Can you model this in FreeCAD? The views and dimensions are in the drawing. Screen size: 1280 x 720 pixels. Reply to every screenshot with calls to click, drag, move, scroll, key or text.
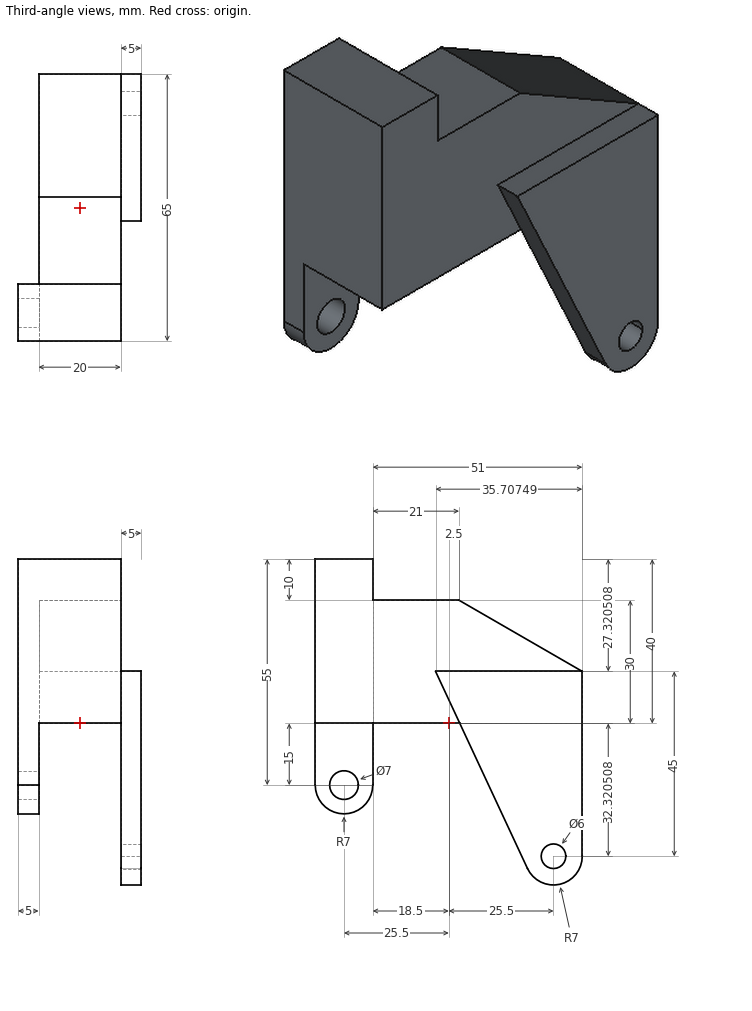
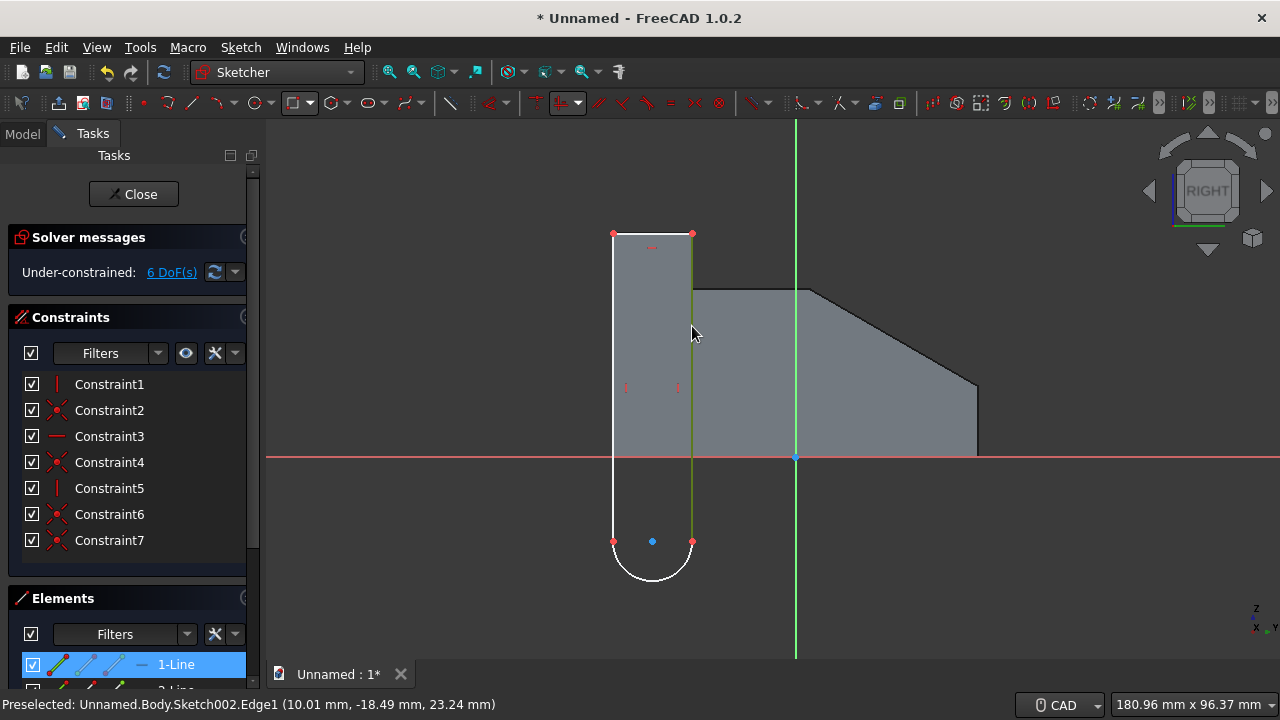
click(629, 574)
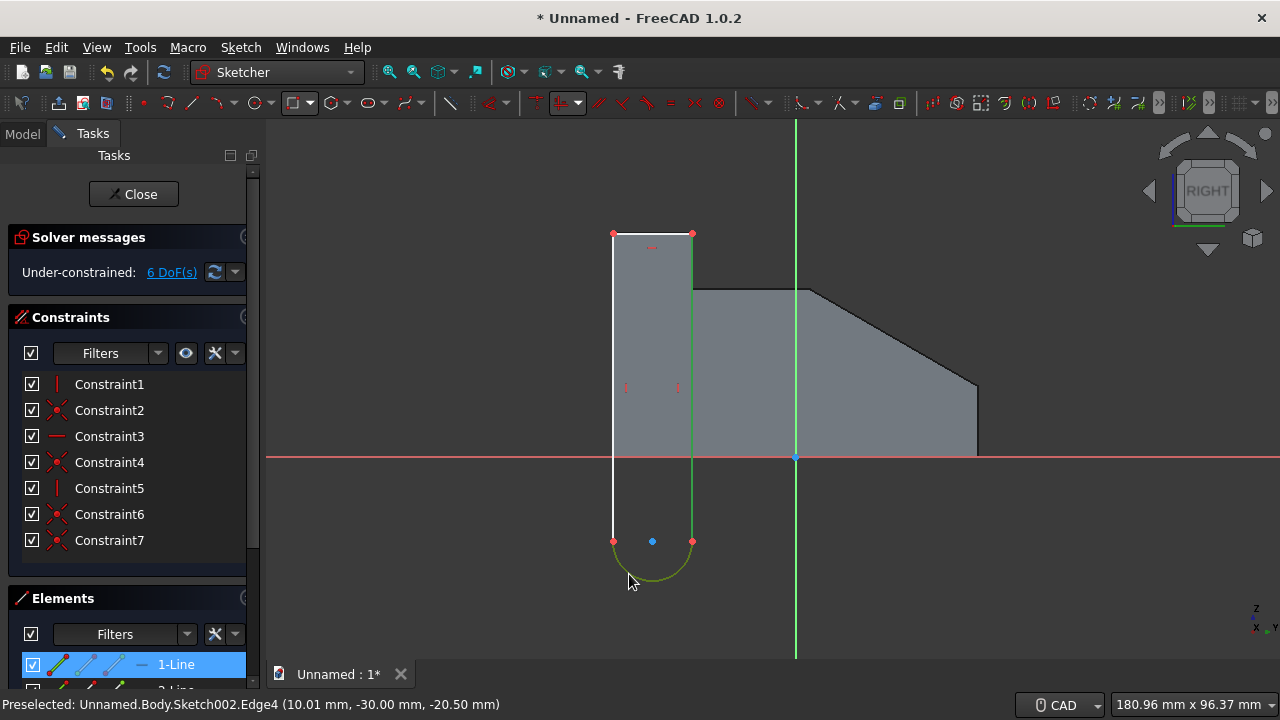
key(t)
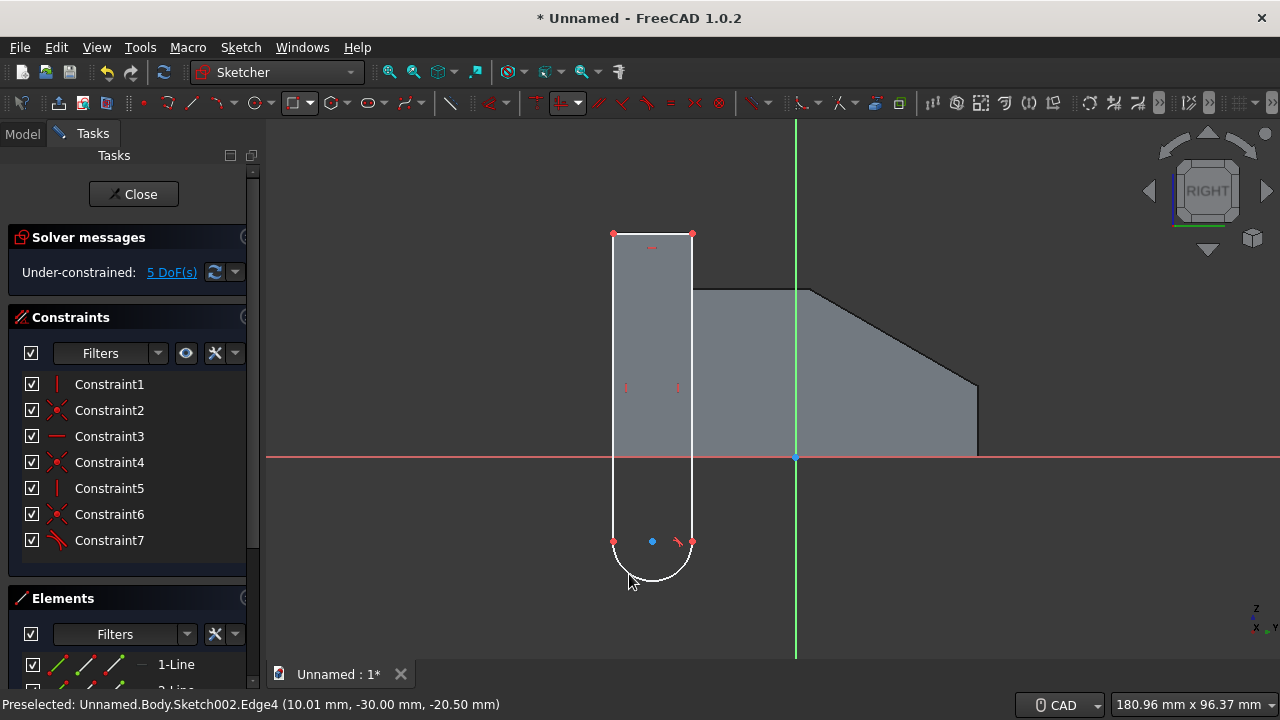
click(613, 326)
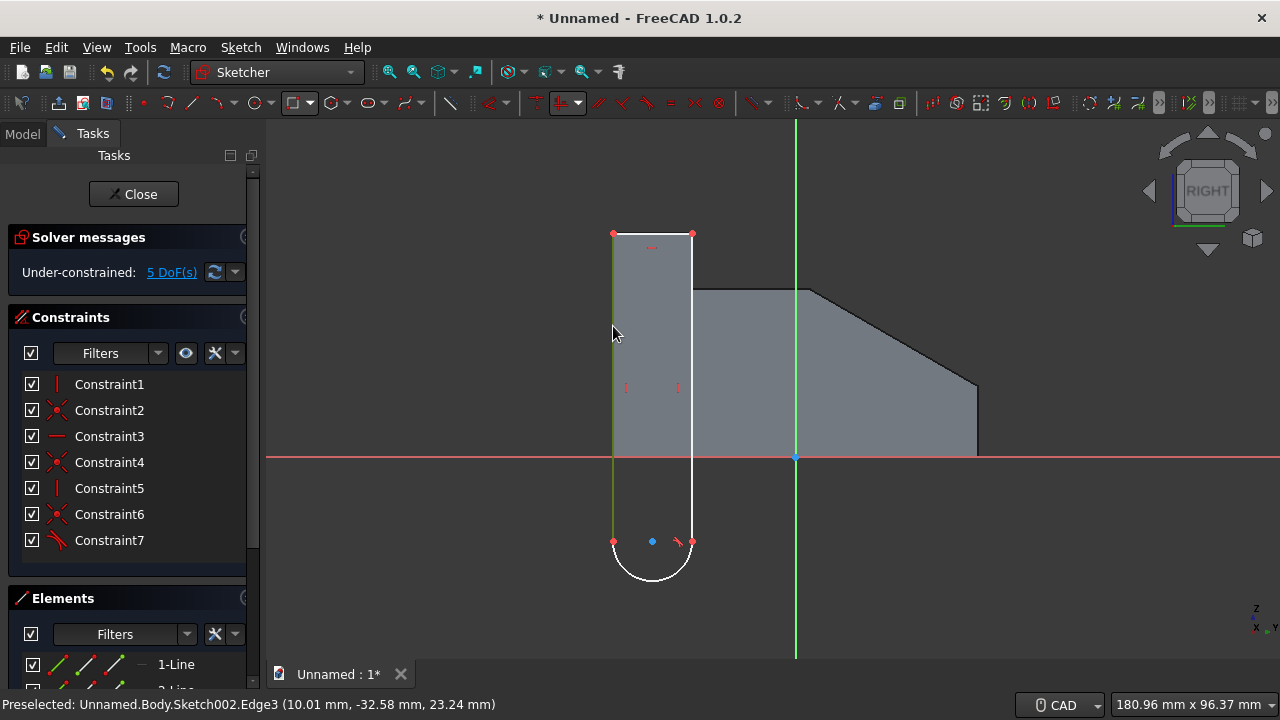
click(630, 574)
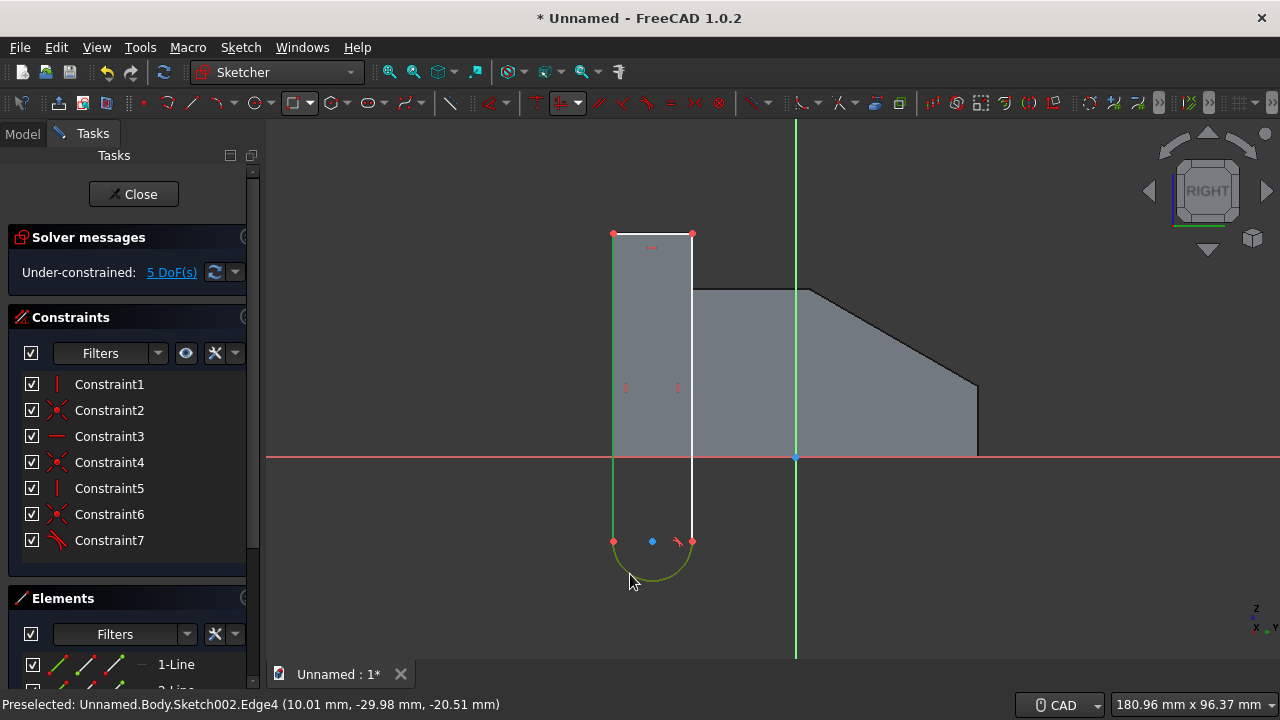
key(t)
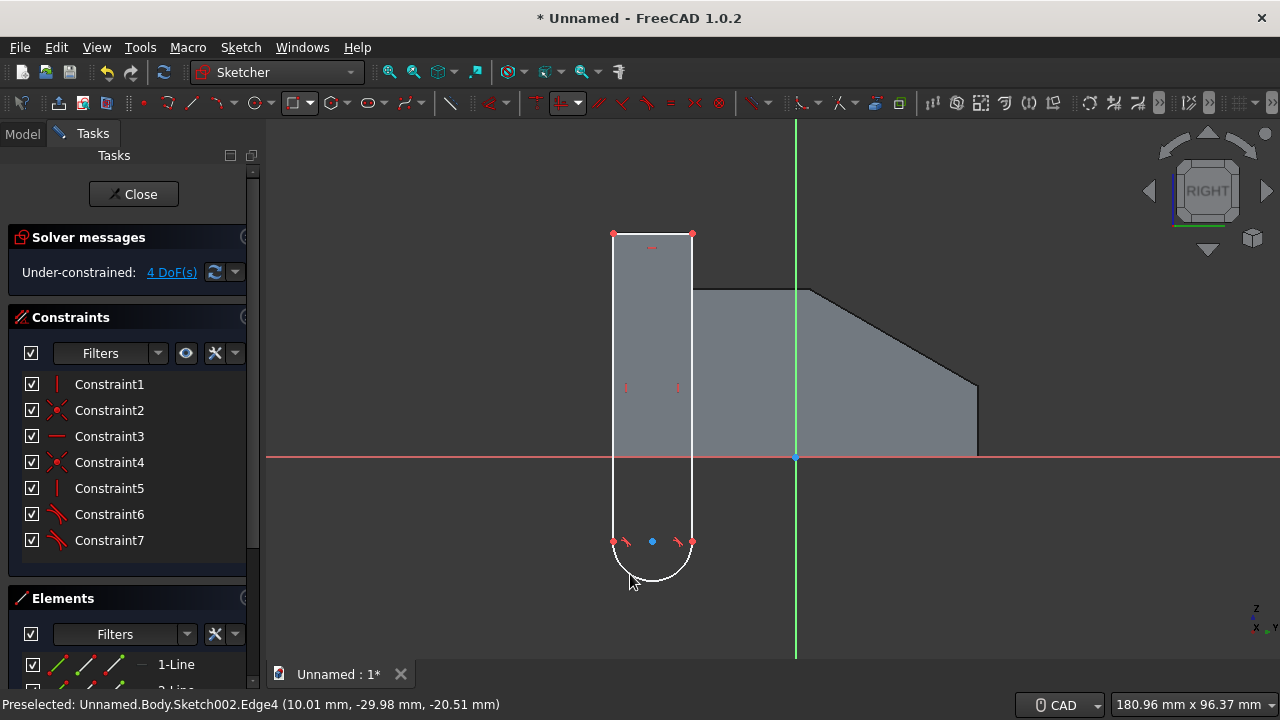
key(d)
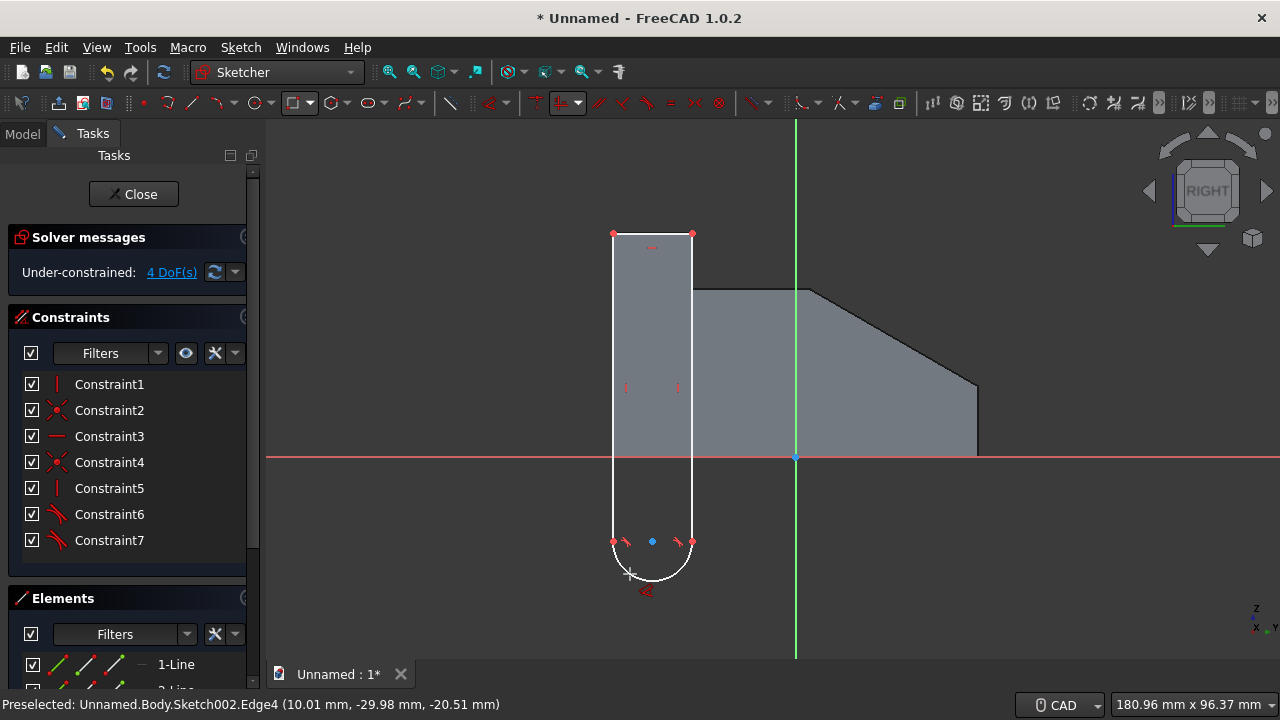
click(629, 573)
click(610, 599)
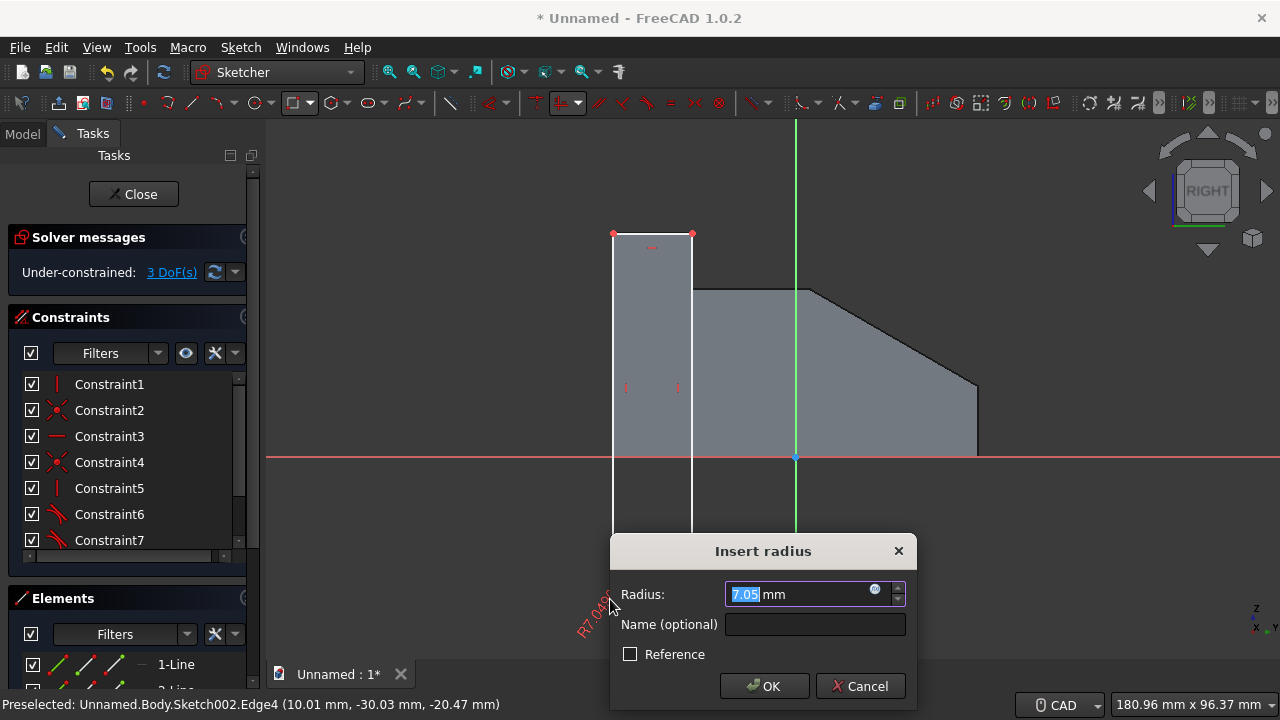
text(7)
key(Return)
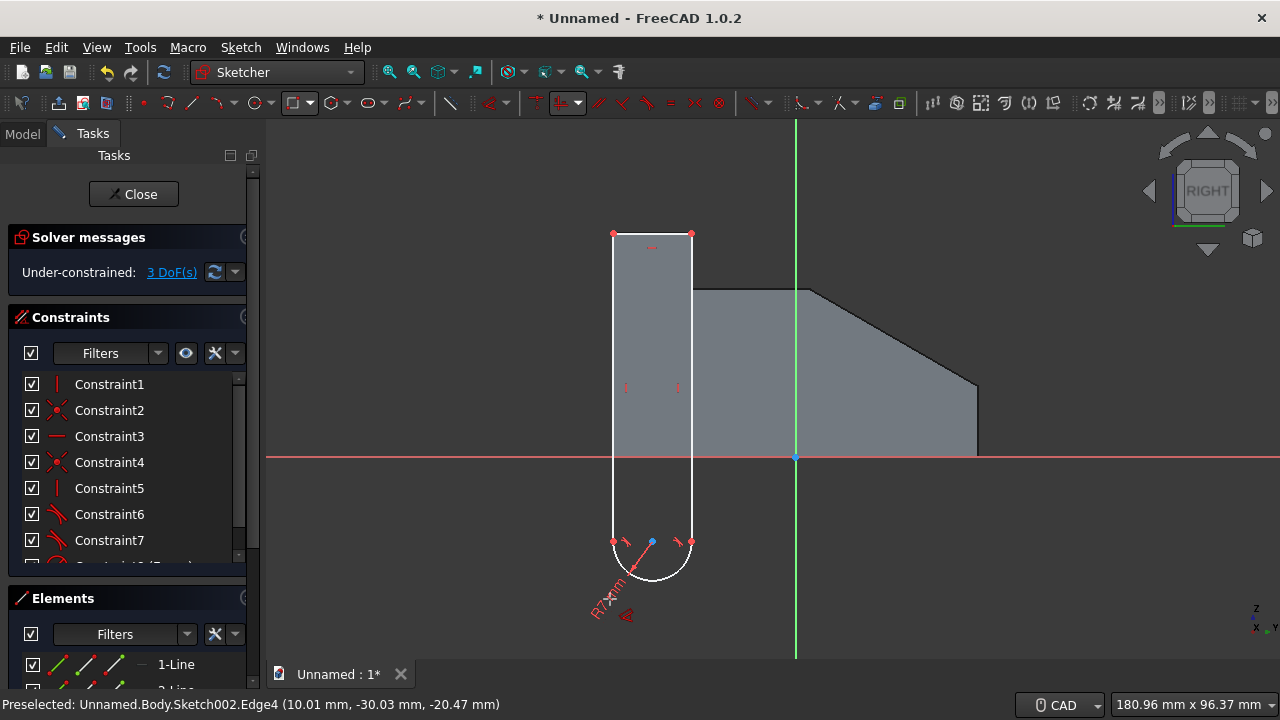
click(692, 326)
click(658, 388)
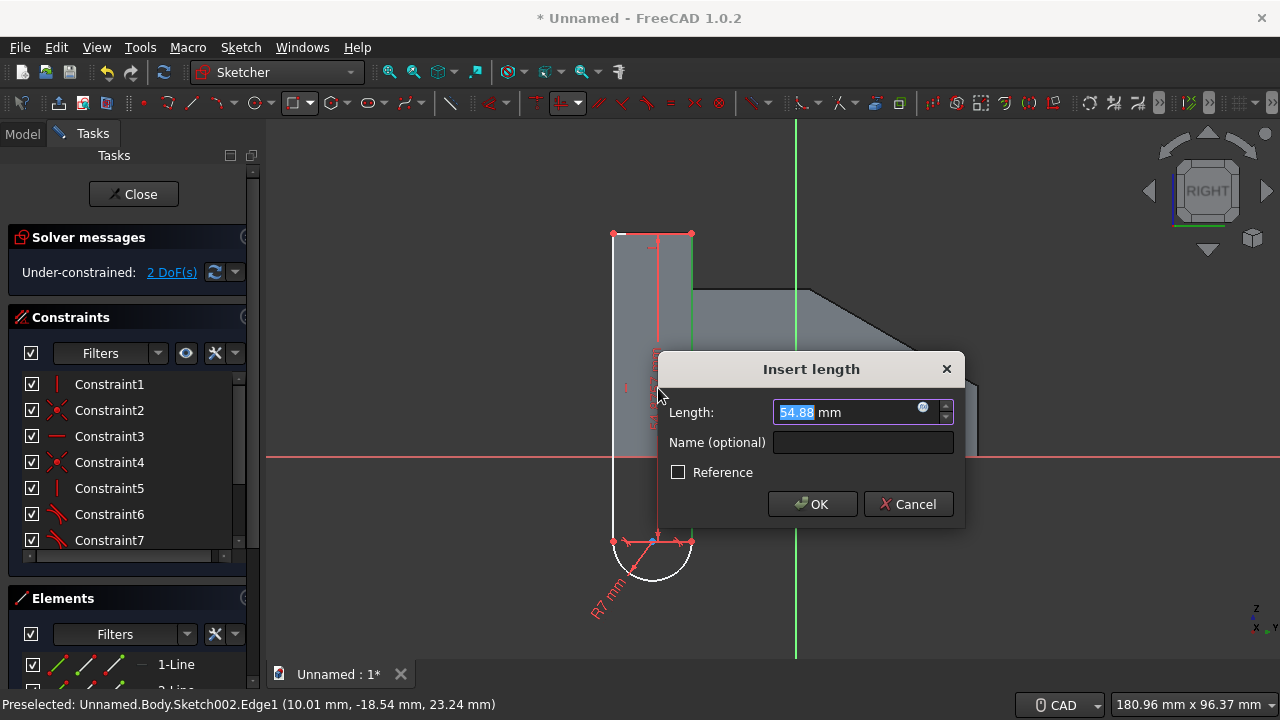
text(55)
key(Return)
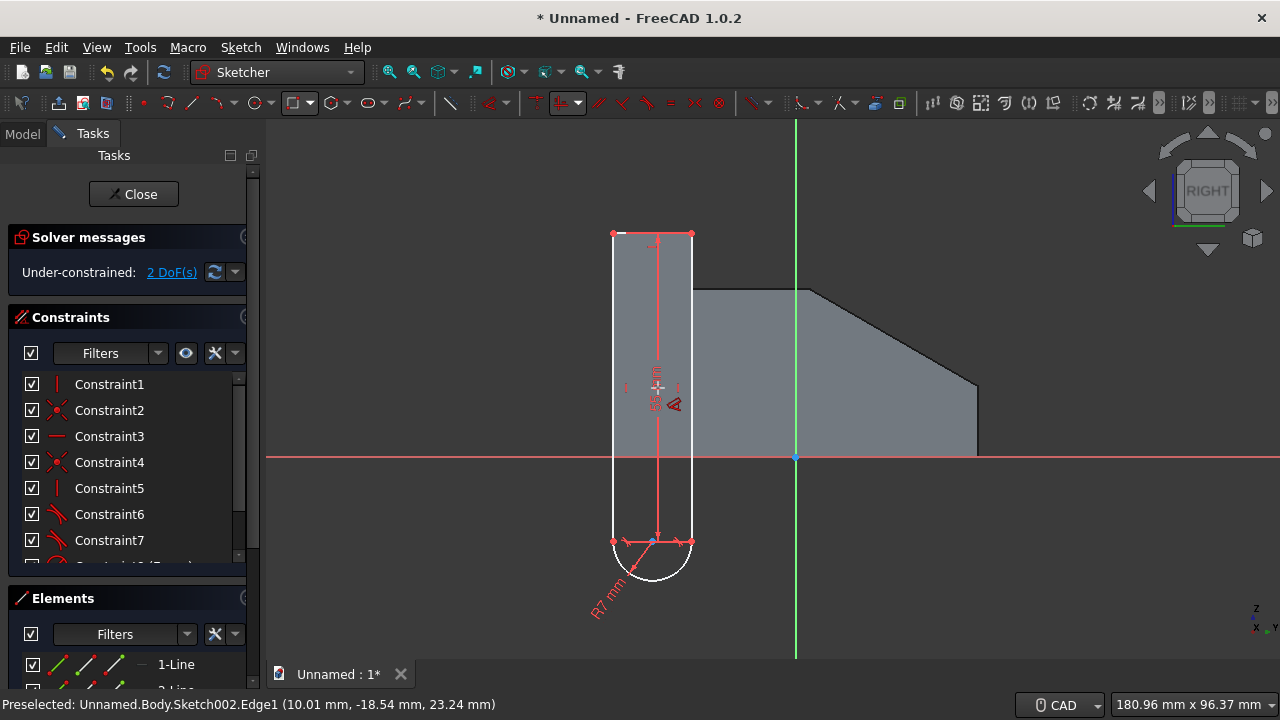
click(692, 541)
click(830, 499)